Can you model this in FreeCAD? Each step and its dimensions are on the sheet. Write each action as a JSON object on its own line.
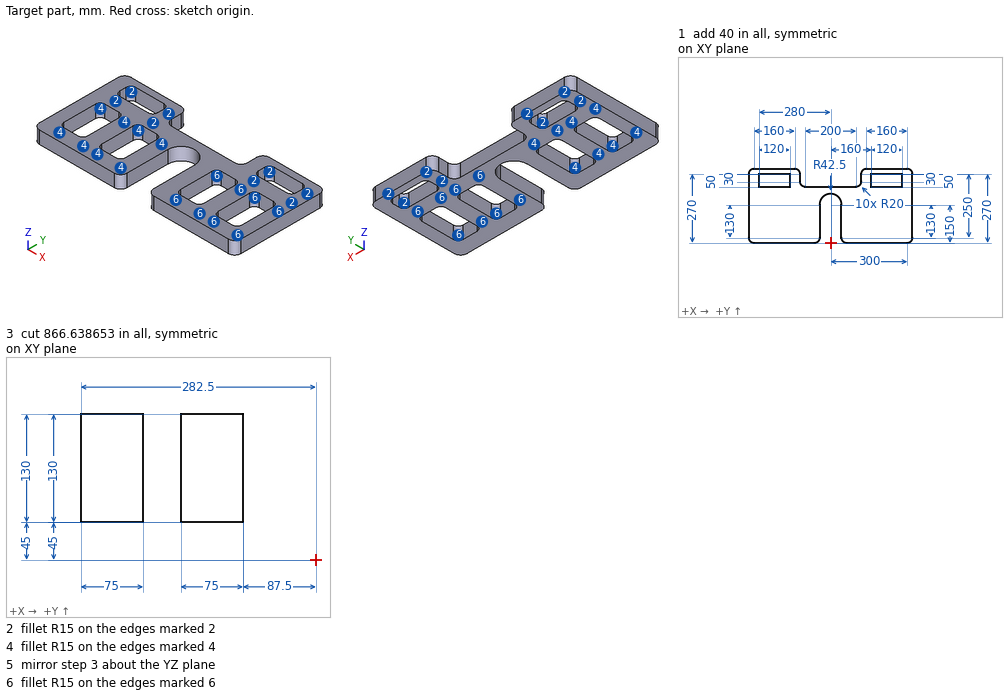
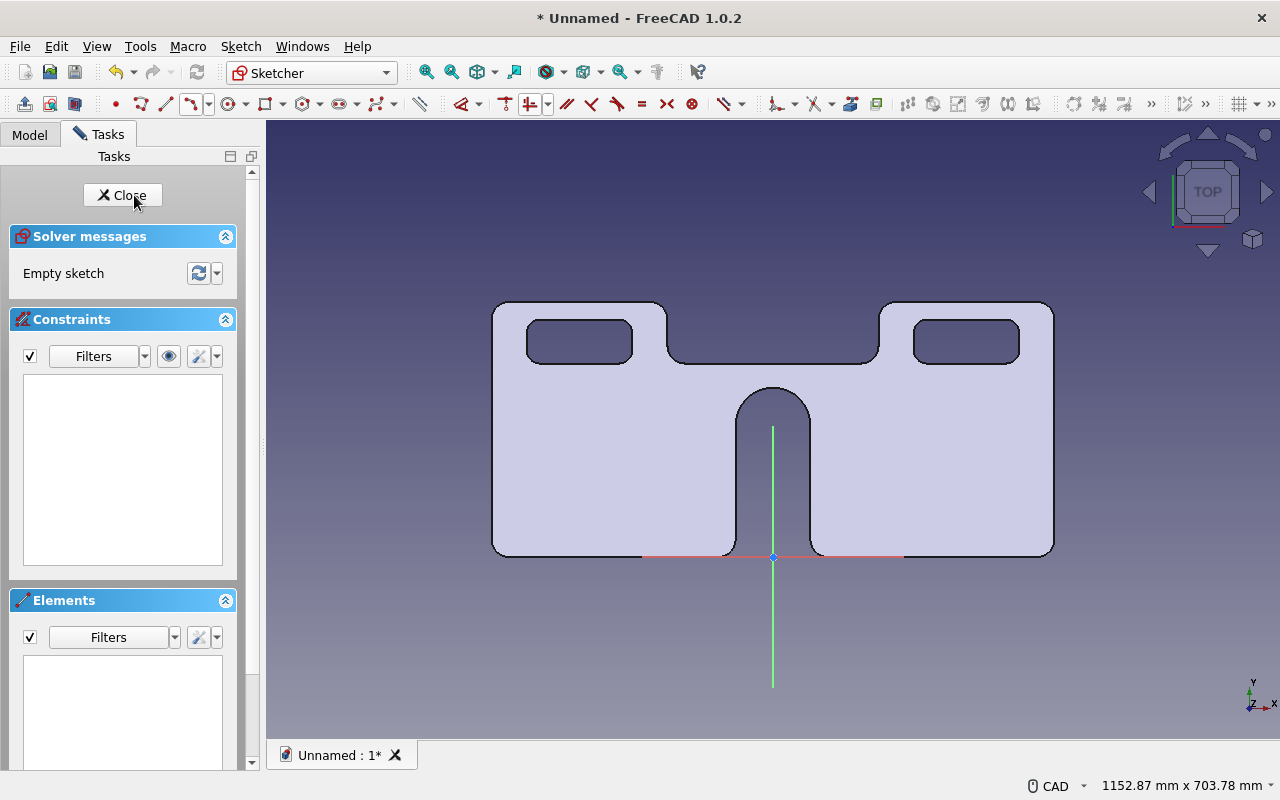
{"action": "scroll", "coordinate": [603, 521], "scroll_direction": "up", "scroll_amount": 4}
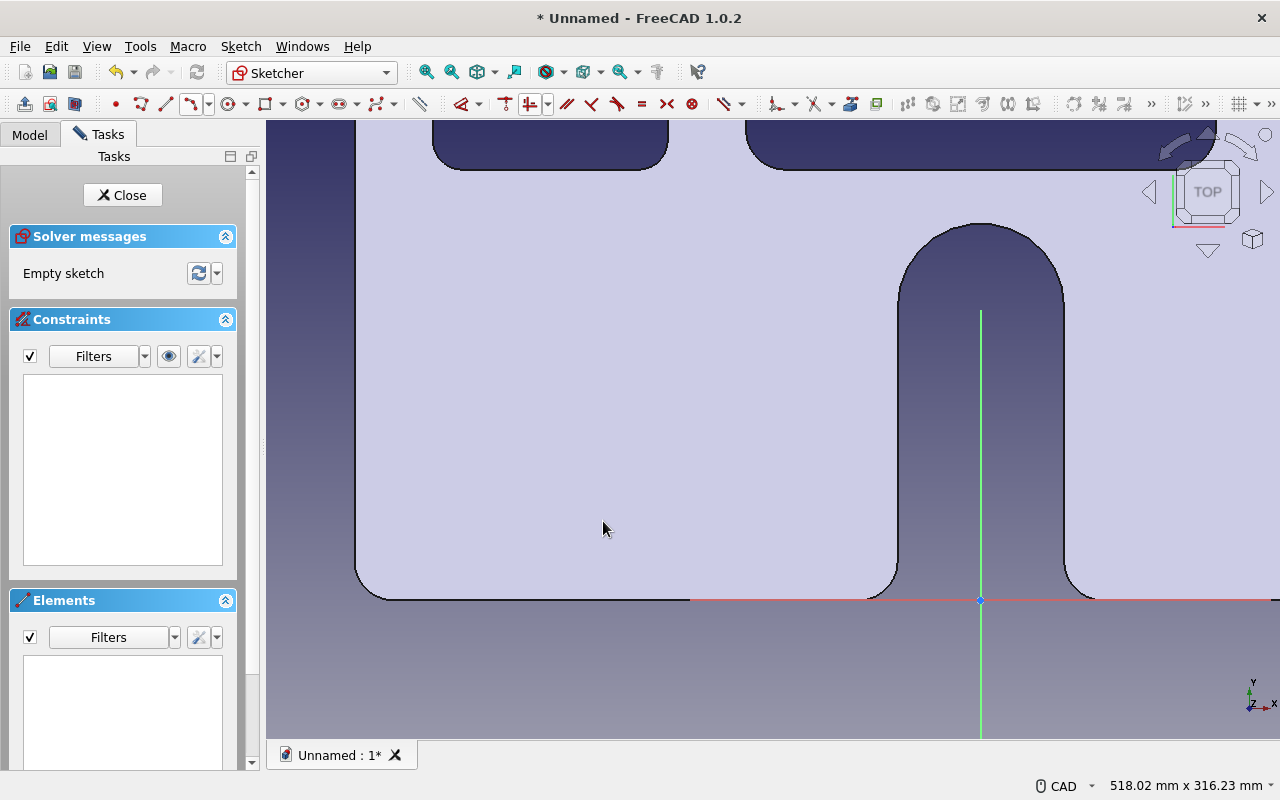
{"action": "key", "text": "g r"}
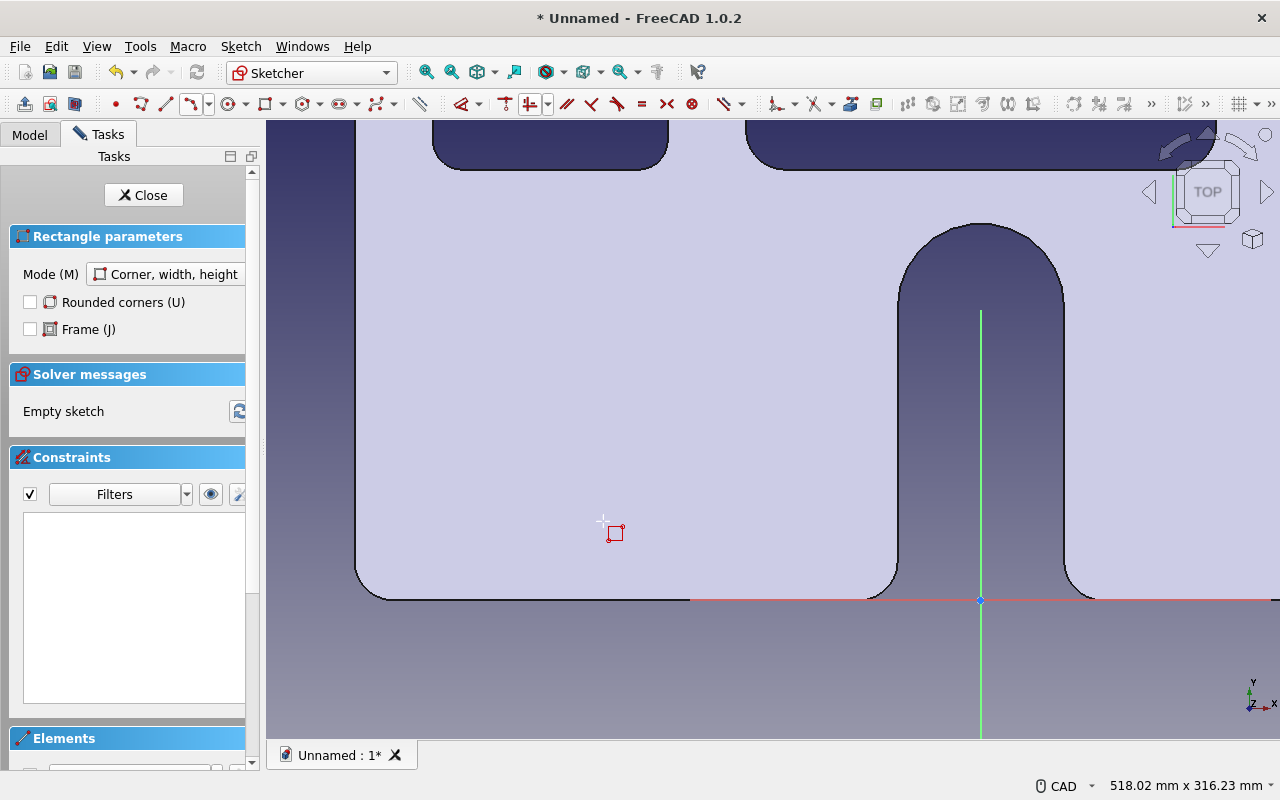
{"action": "left_click", "coordinate": [428, 258]}
{"action": "left_click", "coordinate": [575, 512]}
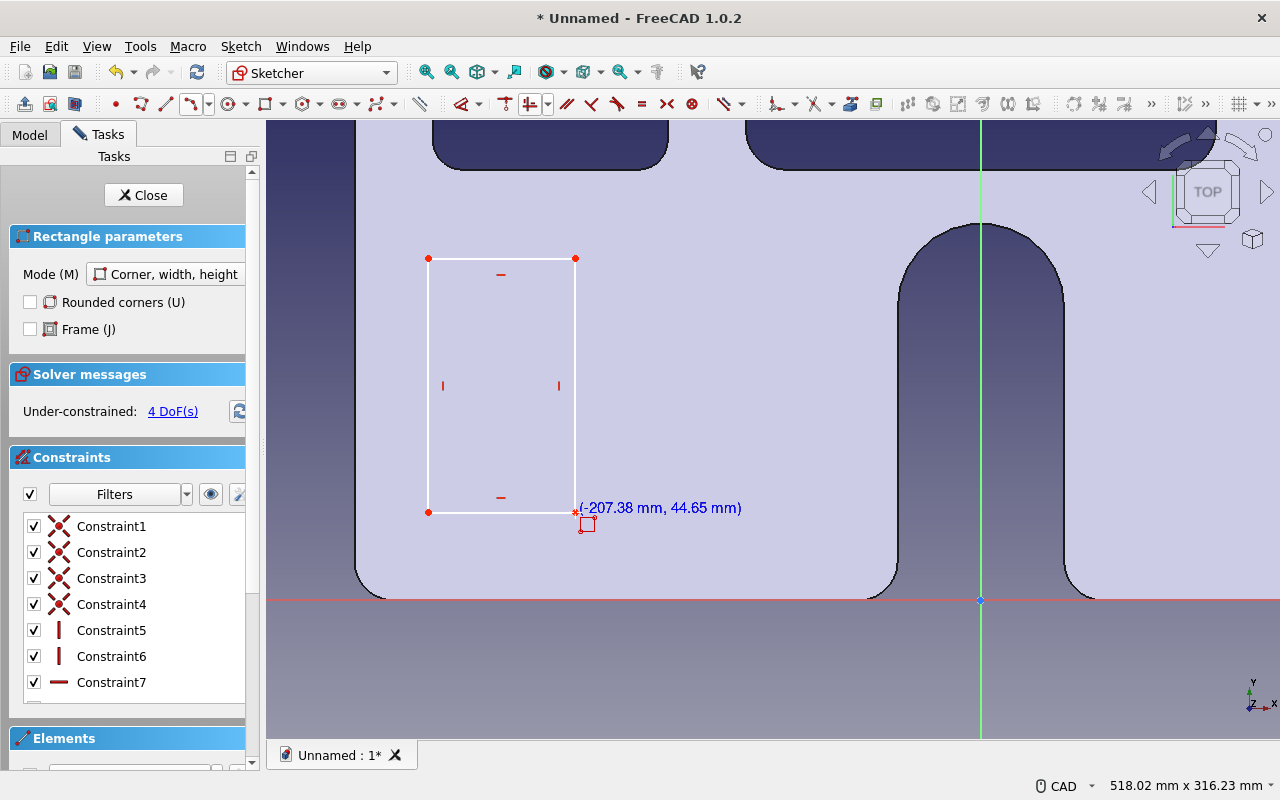
{"action": "left_click", "coordinate": [663, 258]}
{"action": "left_click", "coordinate": [810, 512]}
{"action": "key", "text": "Escape"}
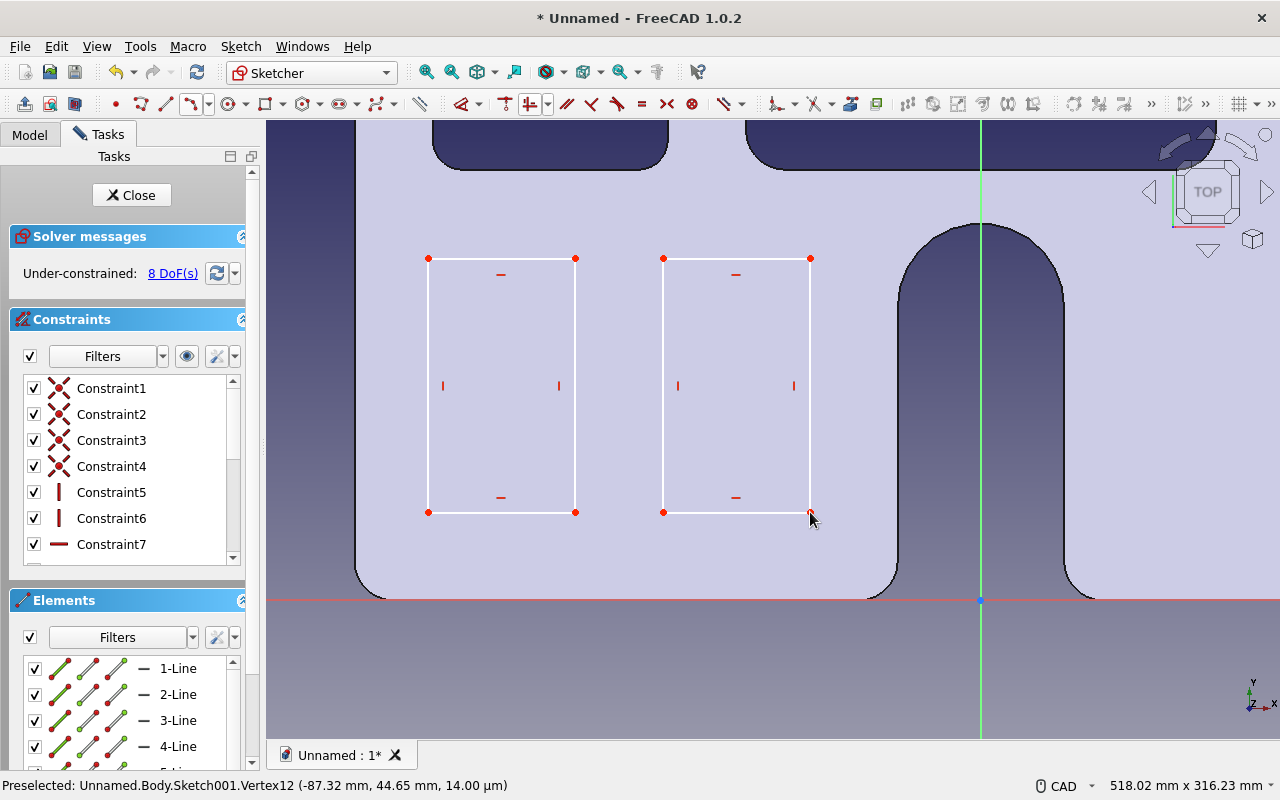
{"action": "left_click", "coordinate": [460, 104]}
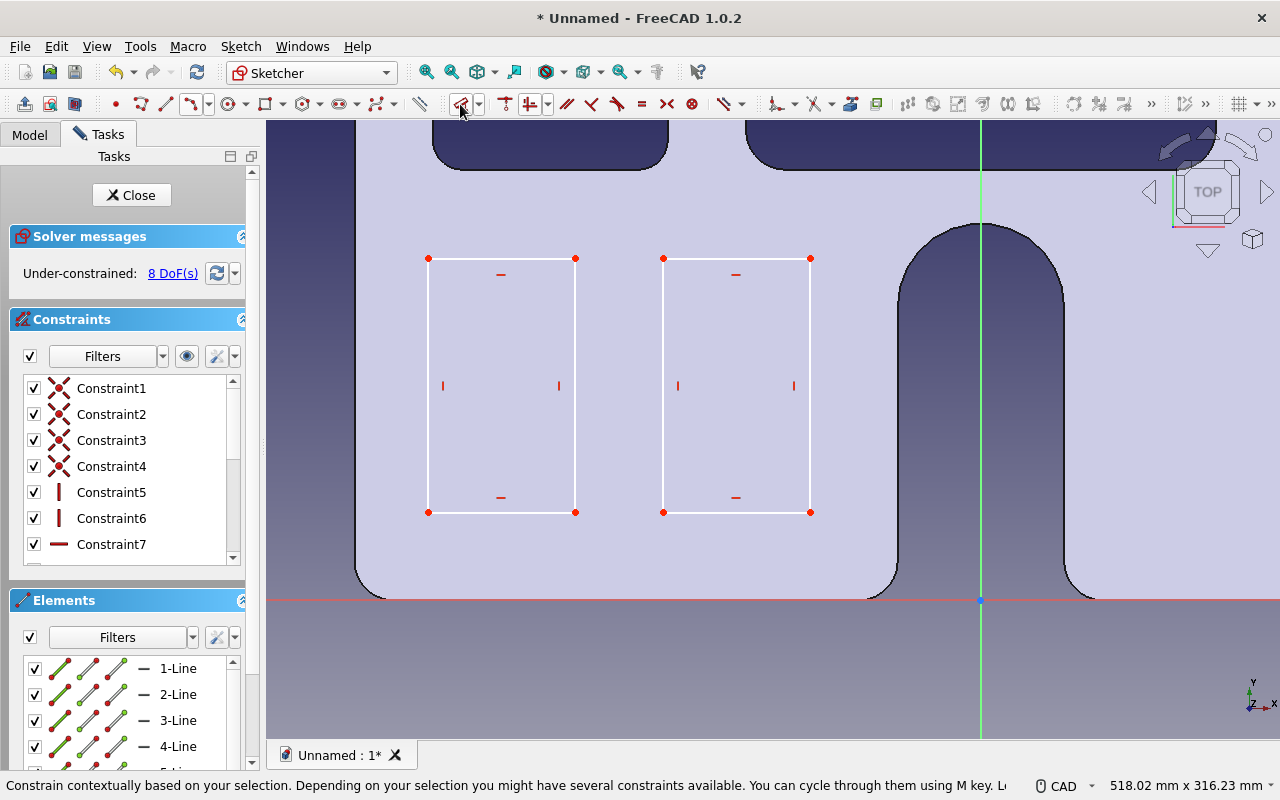
{"action": "left_click", "coordinate": [472, 513]}
{"action": "left_click", "coordinate": [501, 547]}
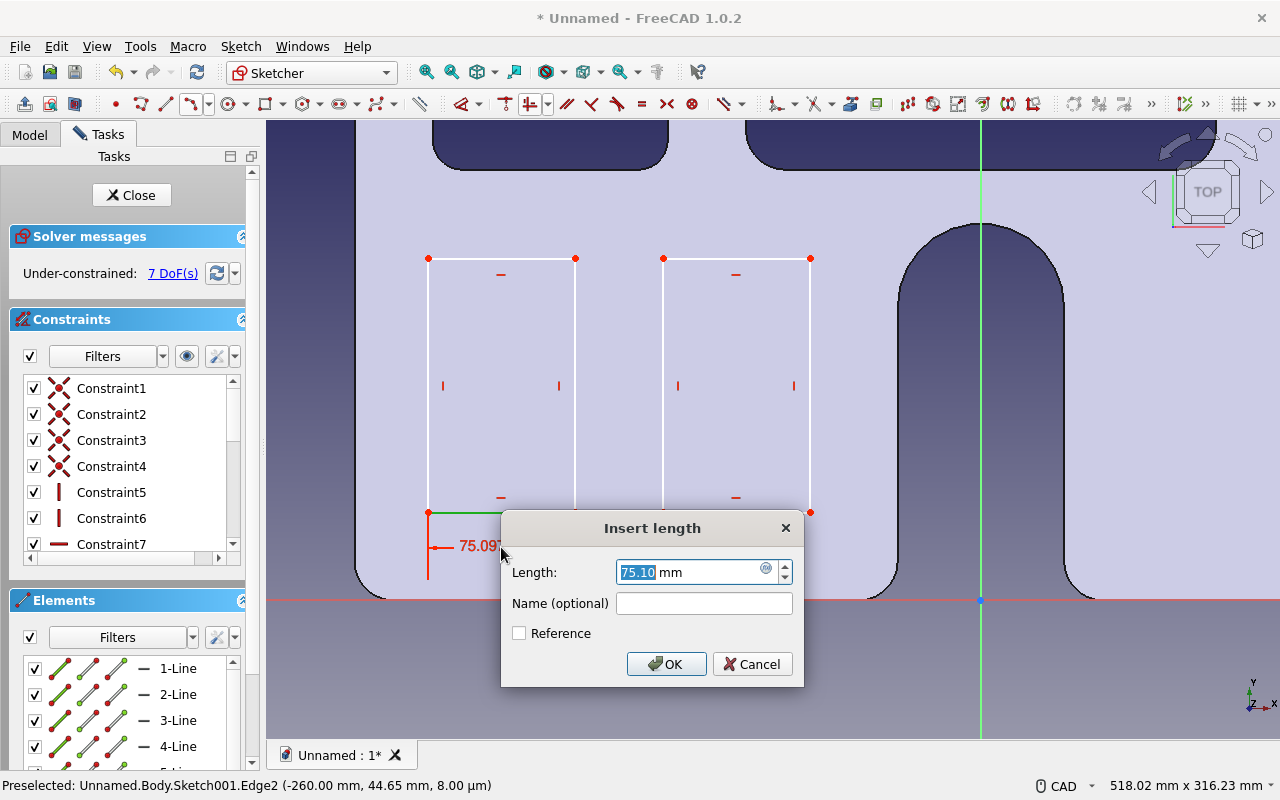
{"action": "type", "text": "75"}
{"action": "key", "text": "Return"}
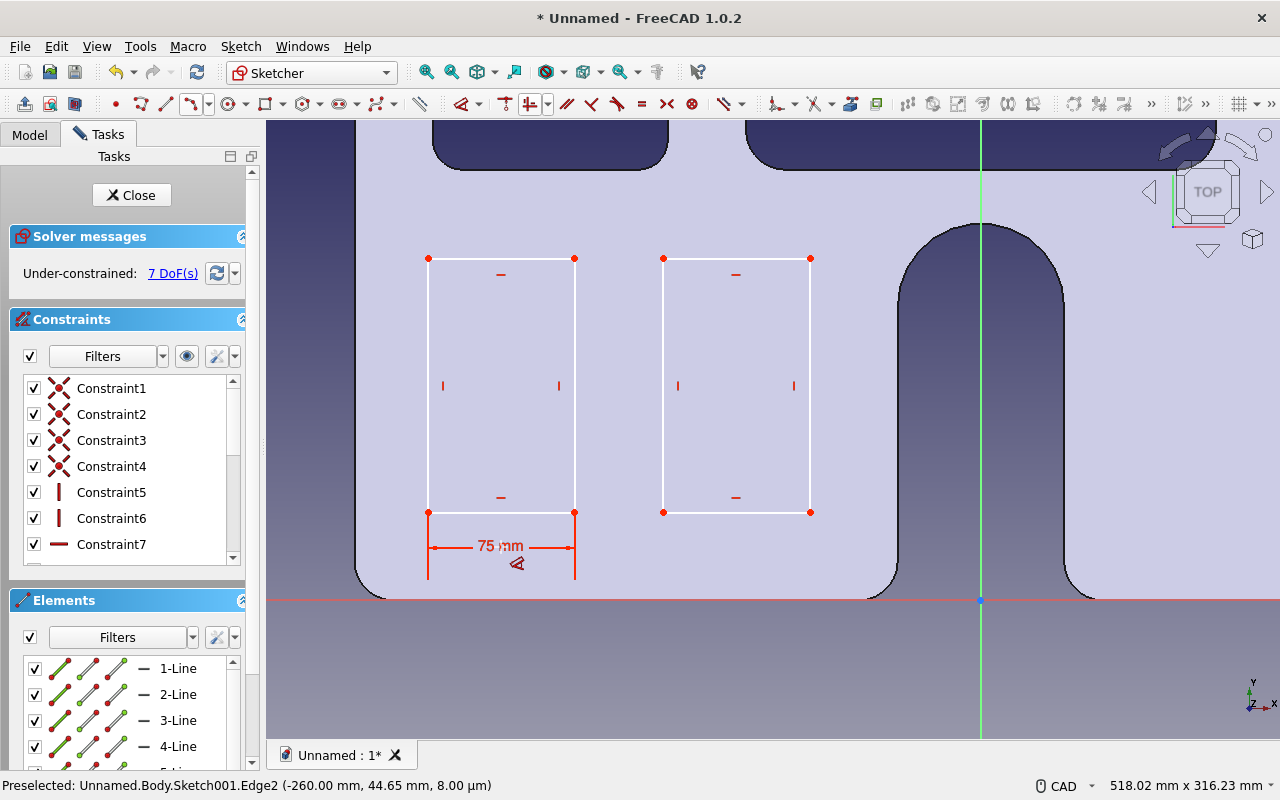
{"action": "left_click", "coordinate": [707, 513]}
{"action": "left_click", "coordinate": [736, 547]}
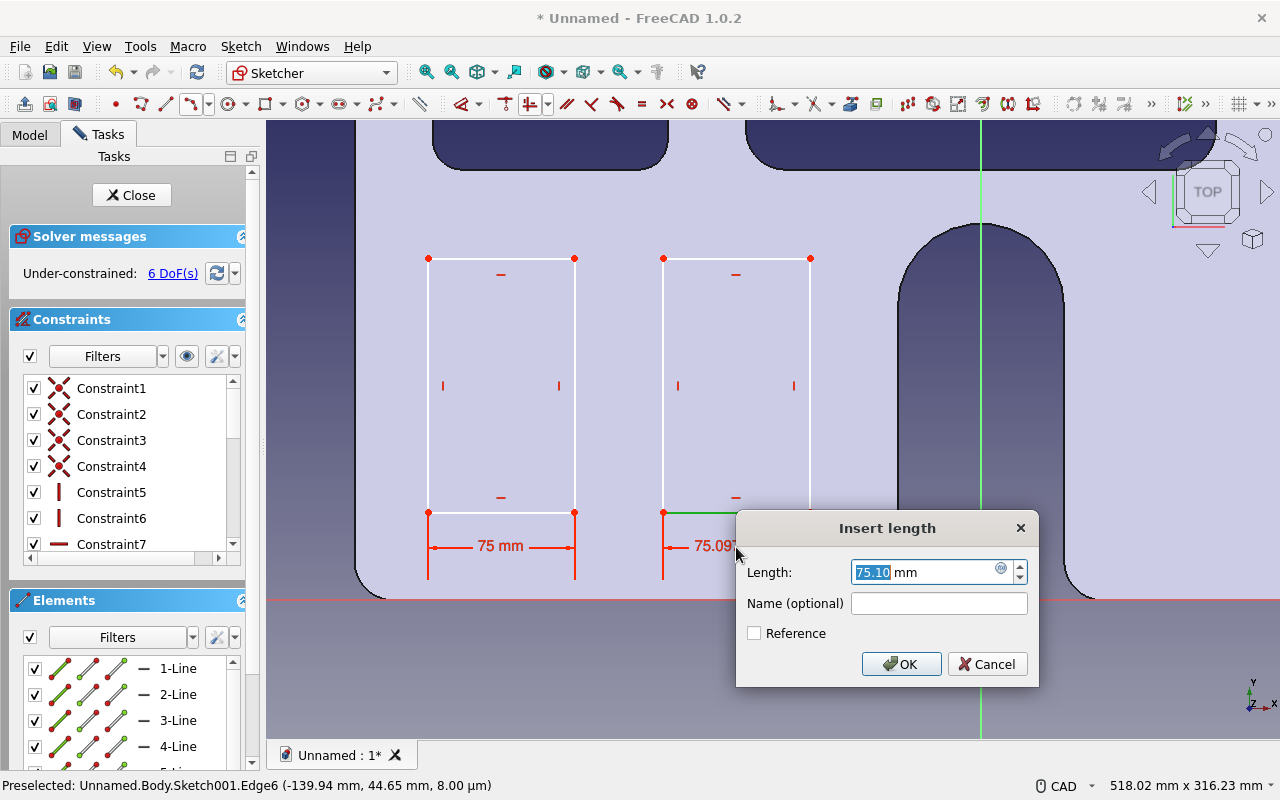
{"action": "type", "text": "75"}
{"action": "key", "text": "Return"}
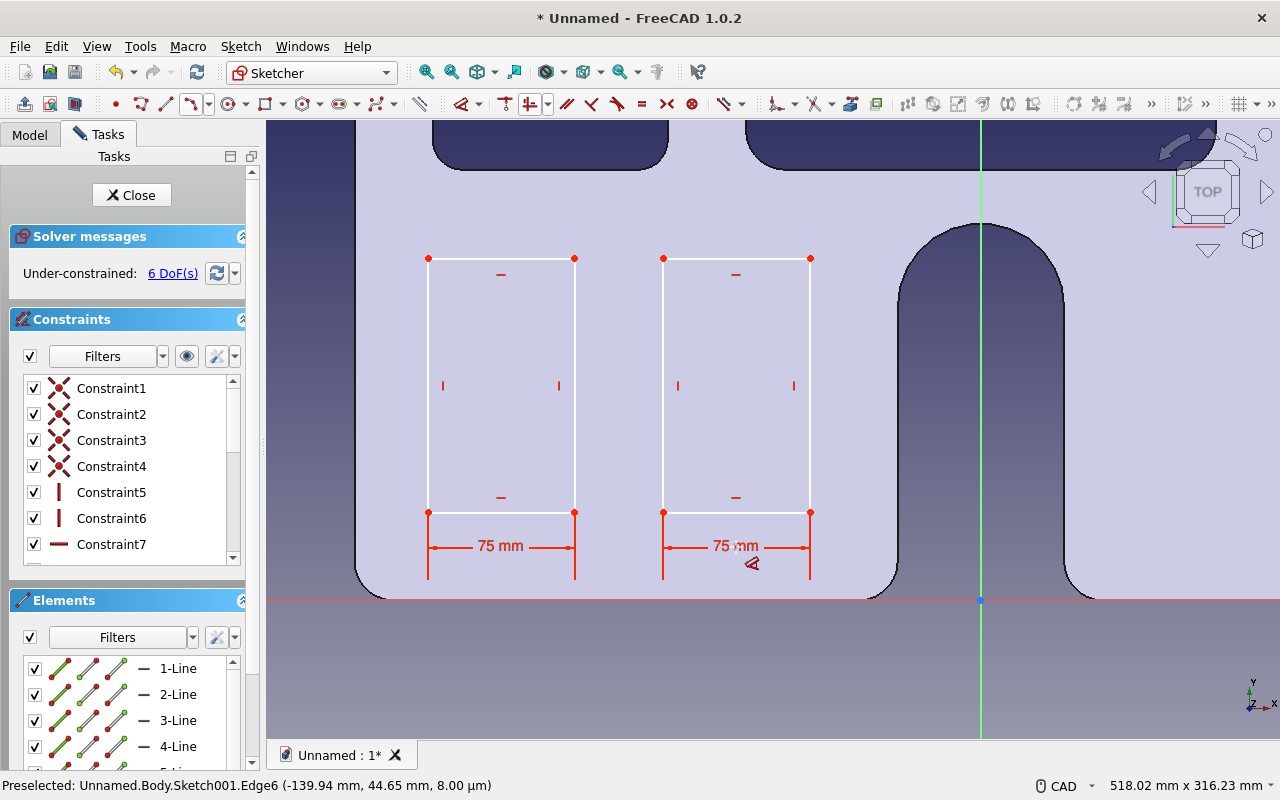
{"action": "left_click", "coordinate": [428, 335]}
{"action": "left_click", "coordinate": [394, 386]}